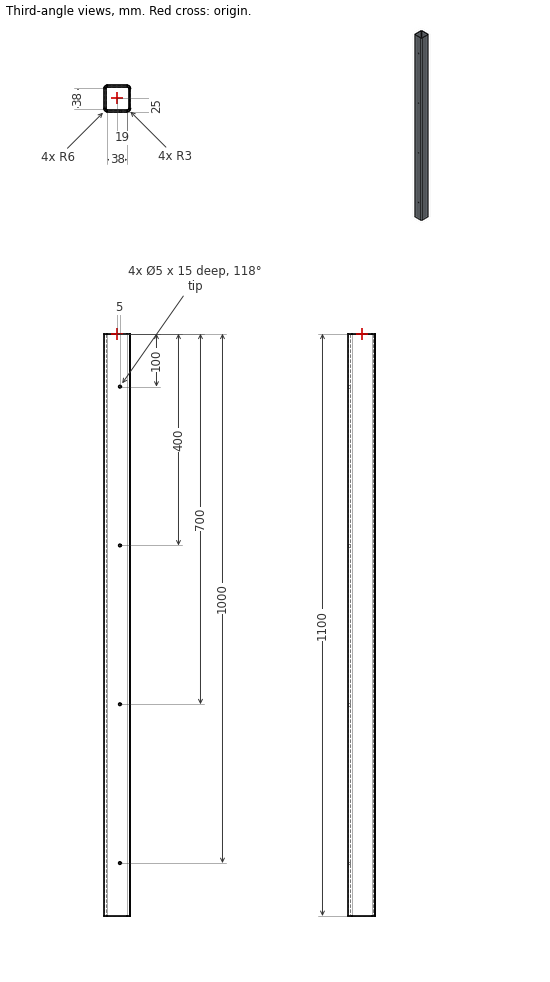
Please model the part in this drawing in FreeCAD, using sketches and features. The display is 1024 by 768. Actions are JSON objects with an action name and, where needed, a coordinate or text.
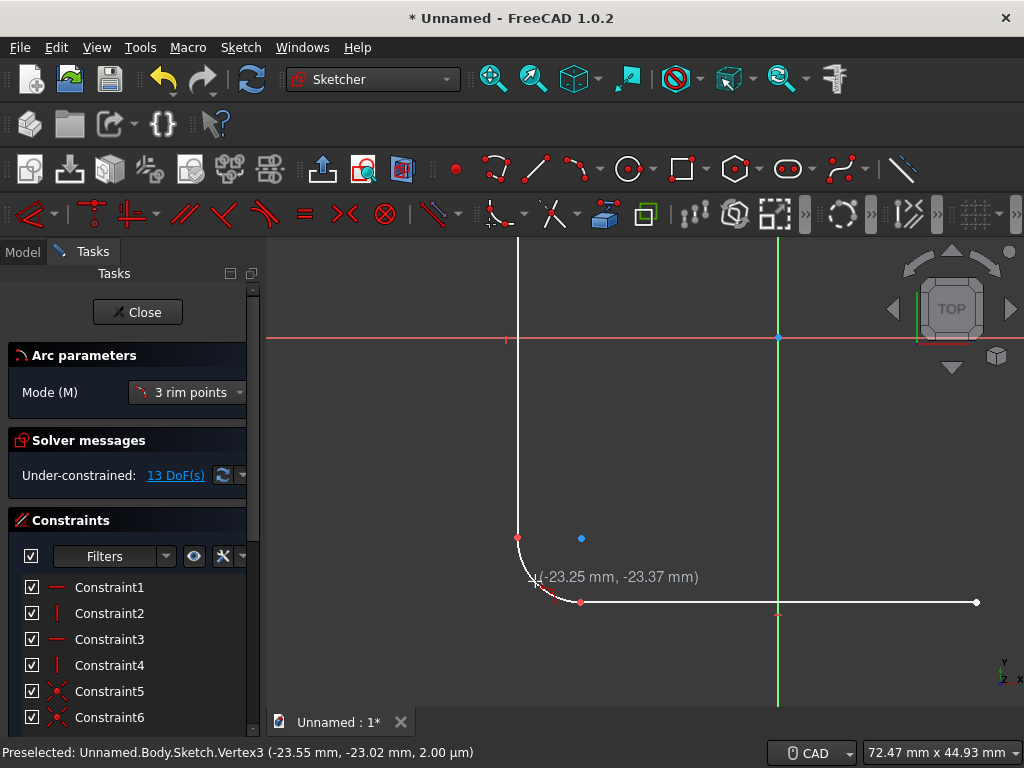
{"action": "scroll", "coordinate": [331, 636], "scroll_direction": "down", "scroll_amount": 3}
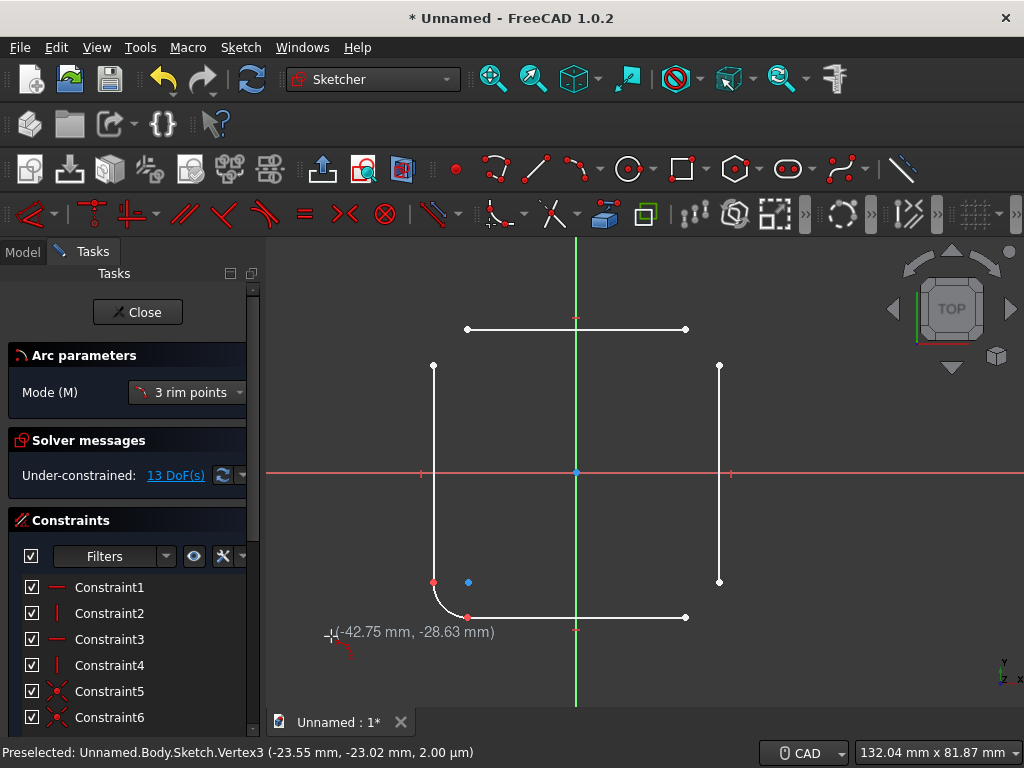
{"action": "left_click", "coordinate": [434, 365]}
{"action": "left_click", "coordinate": [468, 330]}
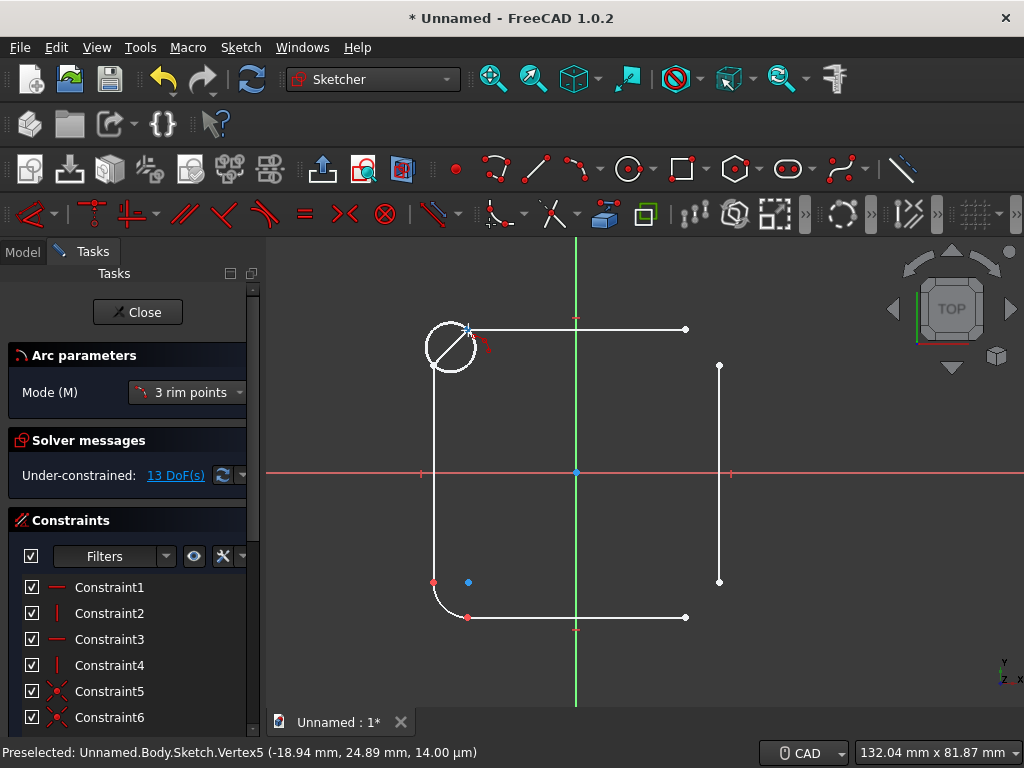
{"action": "scroll", "coordinate": [443, 339], "scroll_direction": "up", "scroll_amount": 3}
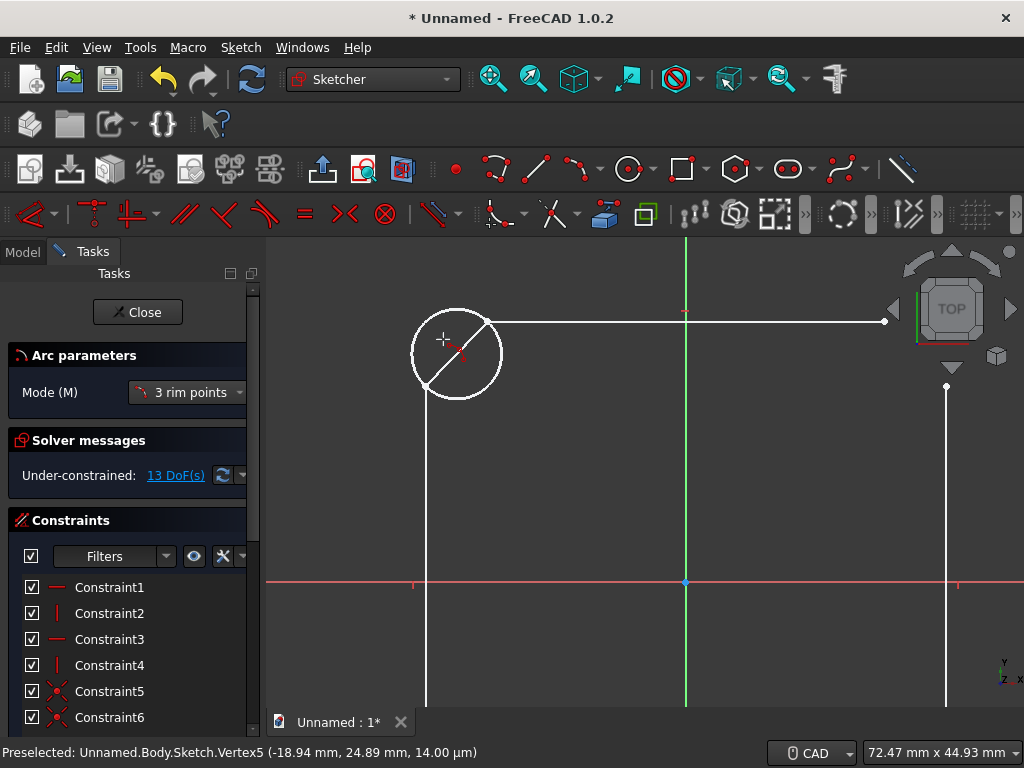
{"action": "left_click", "coordinate": [443, 339]}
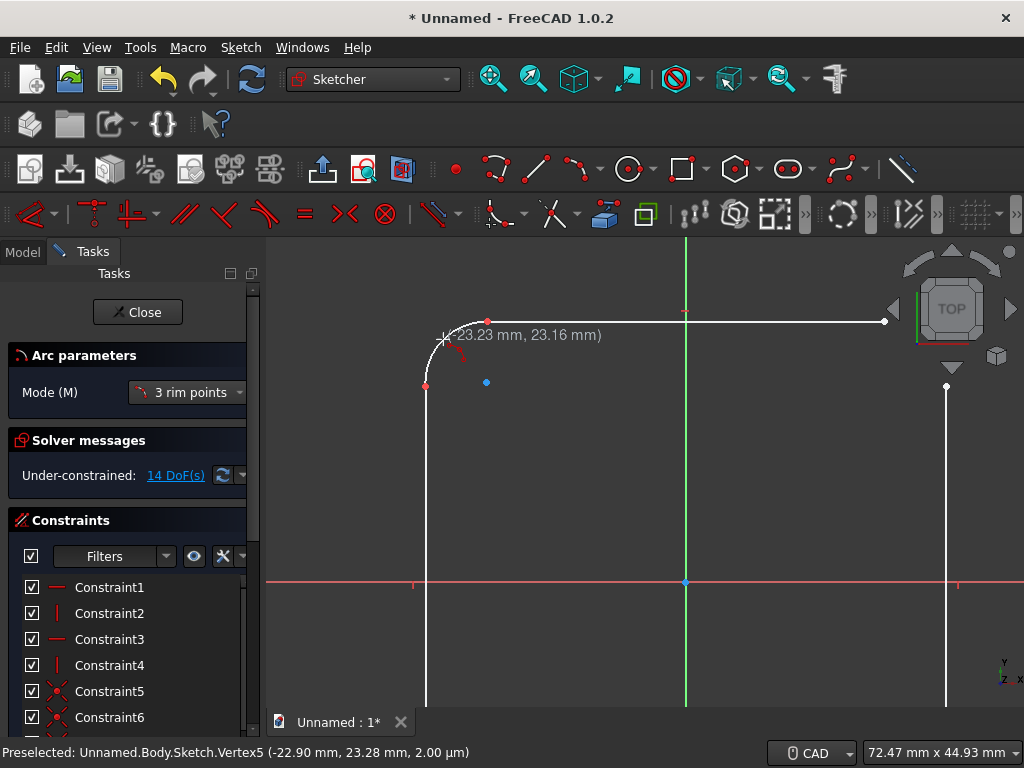
{"action": "scroll", "coordinate": [443, 338], "scroll_direction": "down", "scroll_amount": 3}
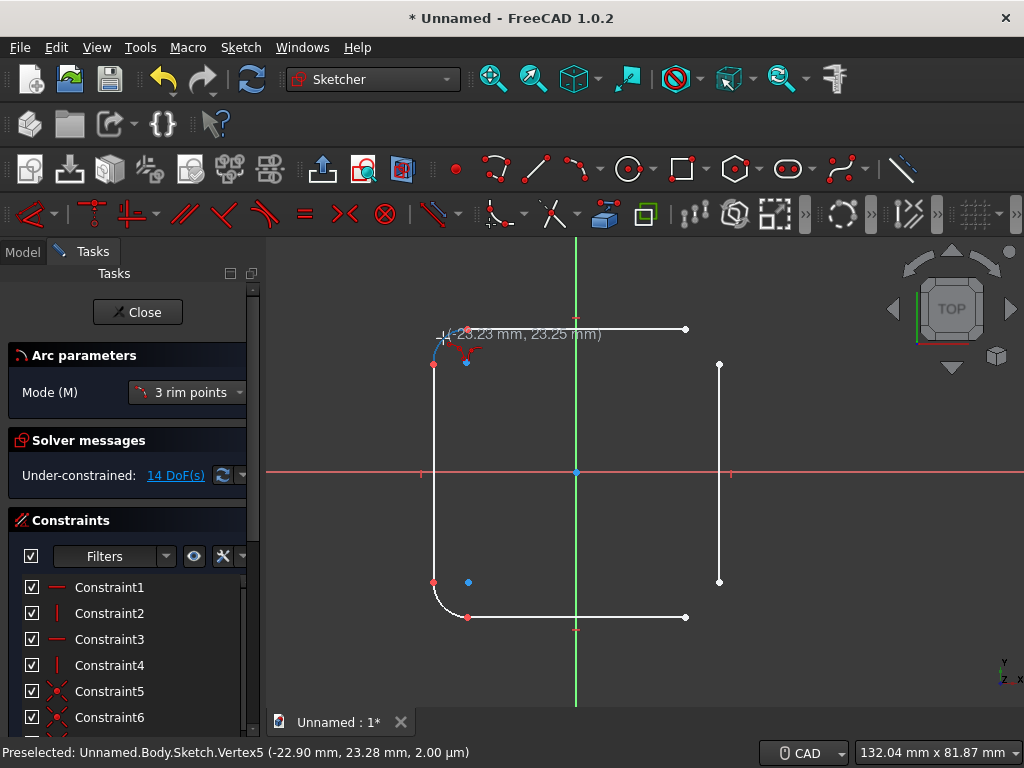
{"action": "left_click", "coordinate": [685, 329]}
{"action": "left_click", "coordinate": [719, 365]}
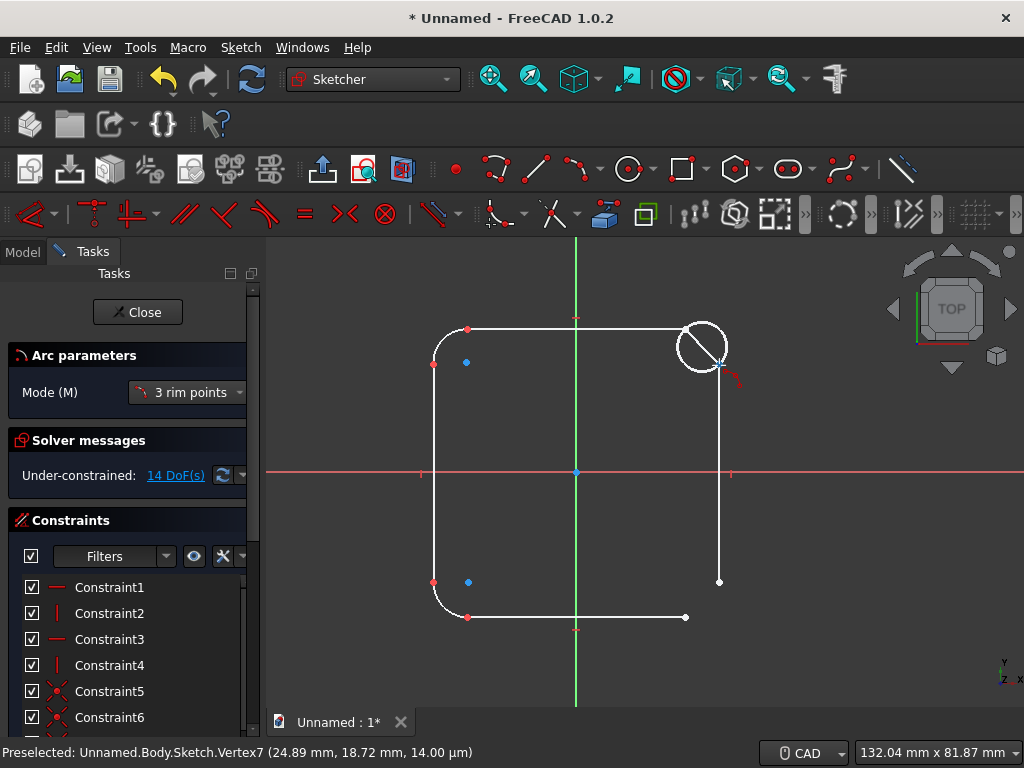
{"action": "scroll", "coordinate": [710, 339], "scroll_direction": "up", "scroll_amount": 3}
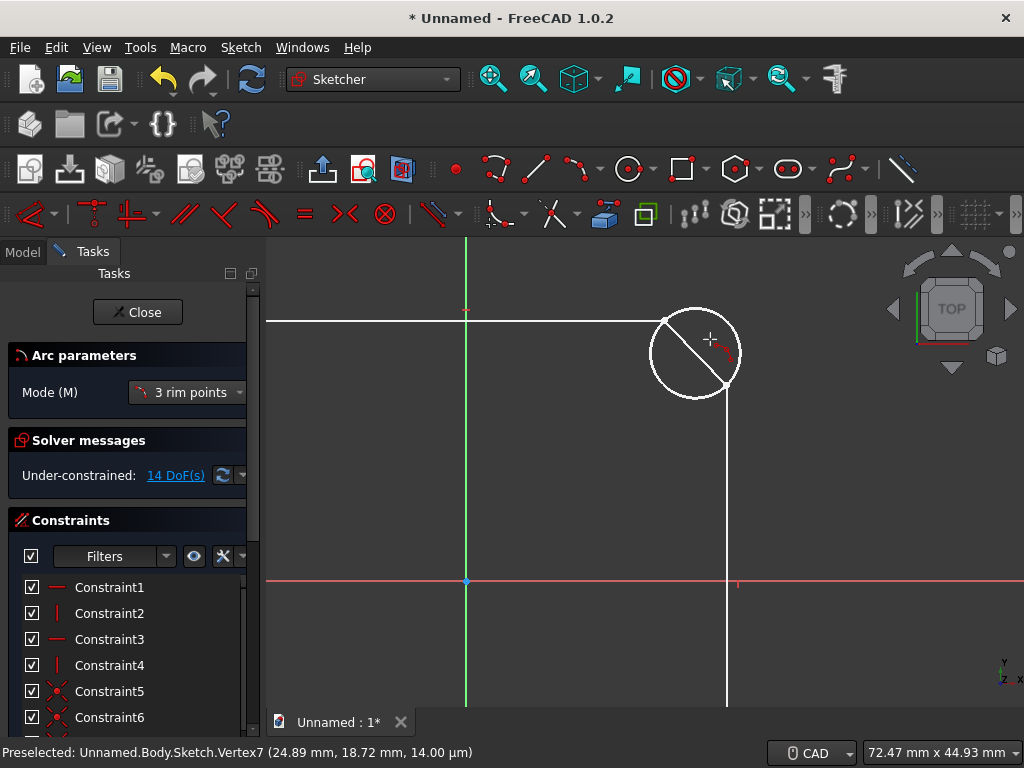
{"action": "left_click", "coordinate": [709, 338]}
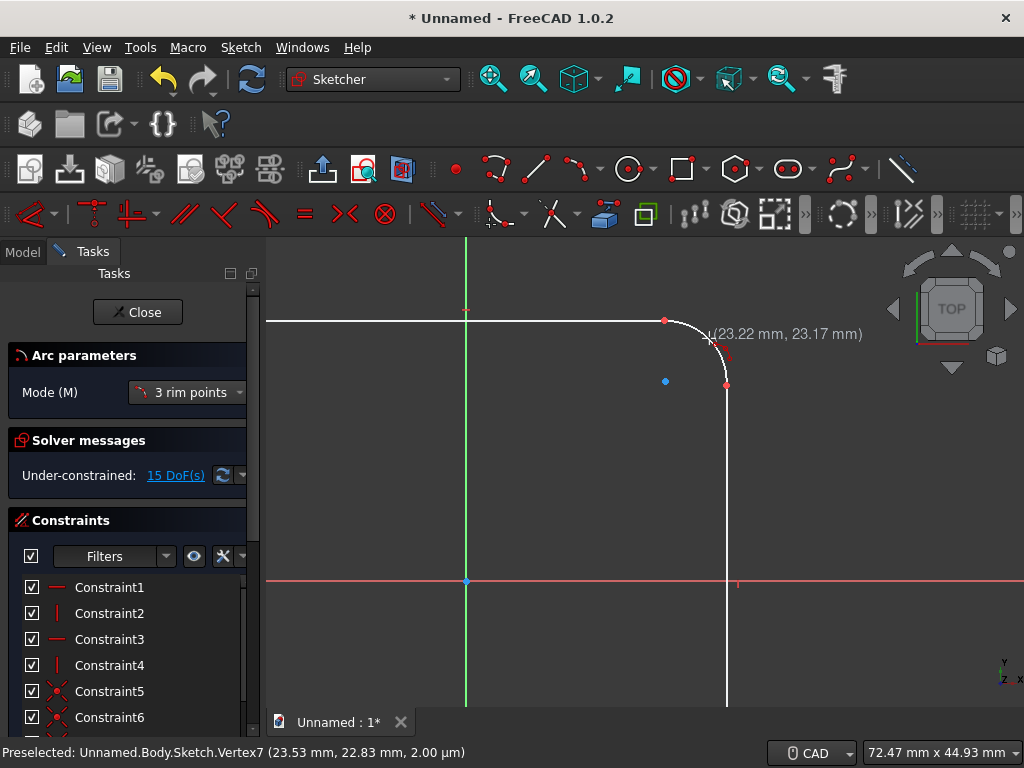
{"action": "scroll", "coordinate": [711, 339], "scroll_direction": "down", "scroll_amount": 3}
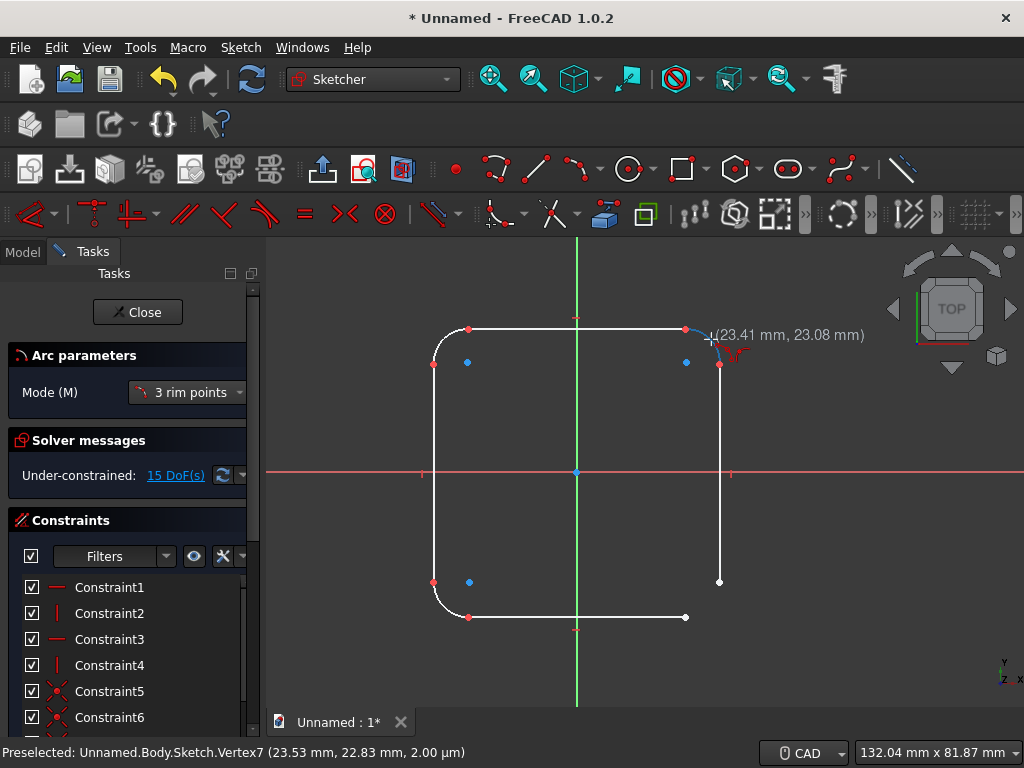
{"action": "left_click", "coordinate": [720, 582]}
{"action": "left_click", "coordinate": [686, 617]}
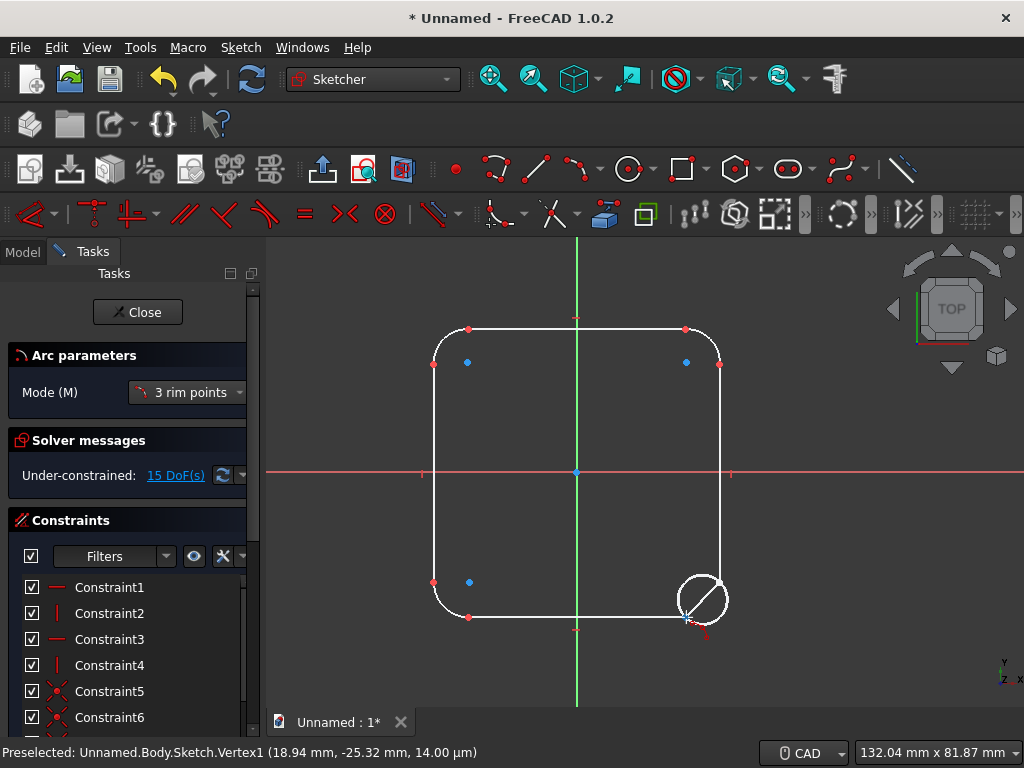
{"action": "scroll", "coordinate": [710, 606], "scroll_direction": "up", "scroll_amount": 3}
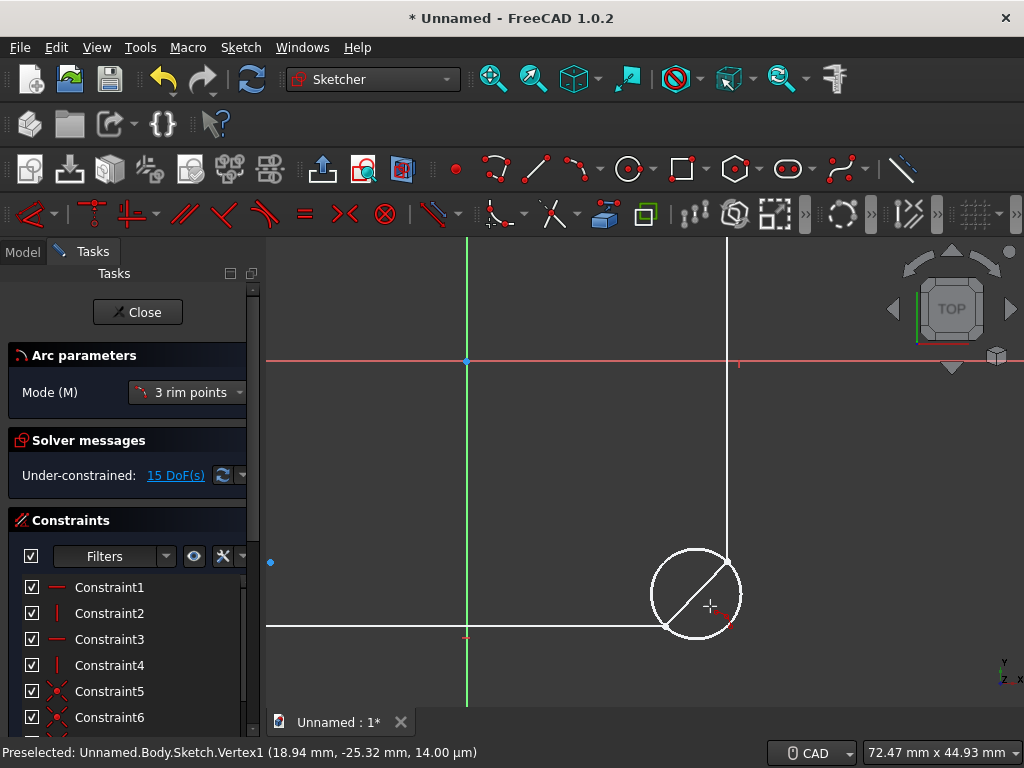
{"action": "left_click", "coordinate": [710, 605]}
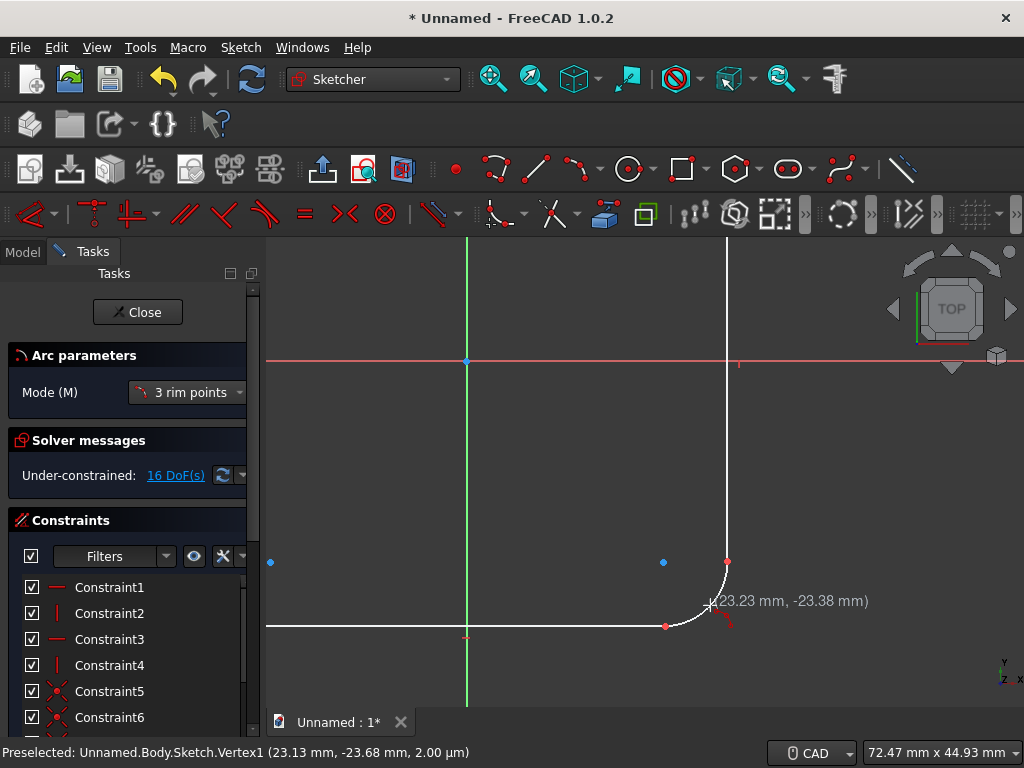
{"action": "key", "text": "g l"}